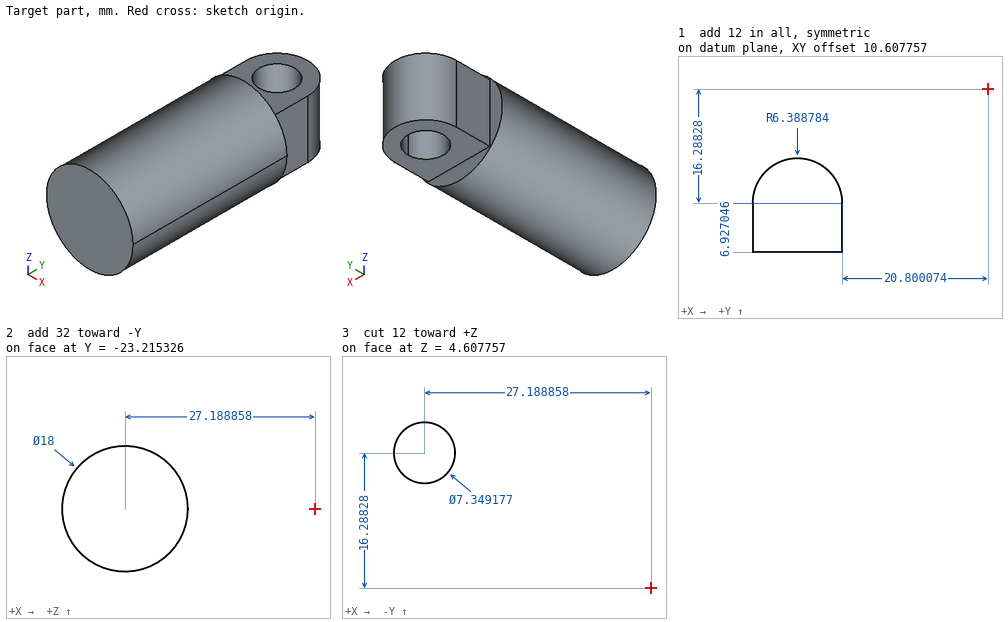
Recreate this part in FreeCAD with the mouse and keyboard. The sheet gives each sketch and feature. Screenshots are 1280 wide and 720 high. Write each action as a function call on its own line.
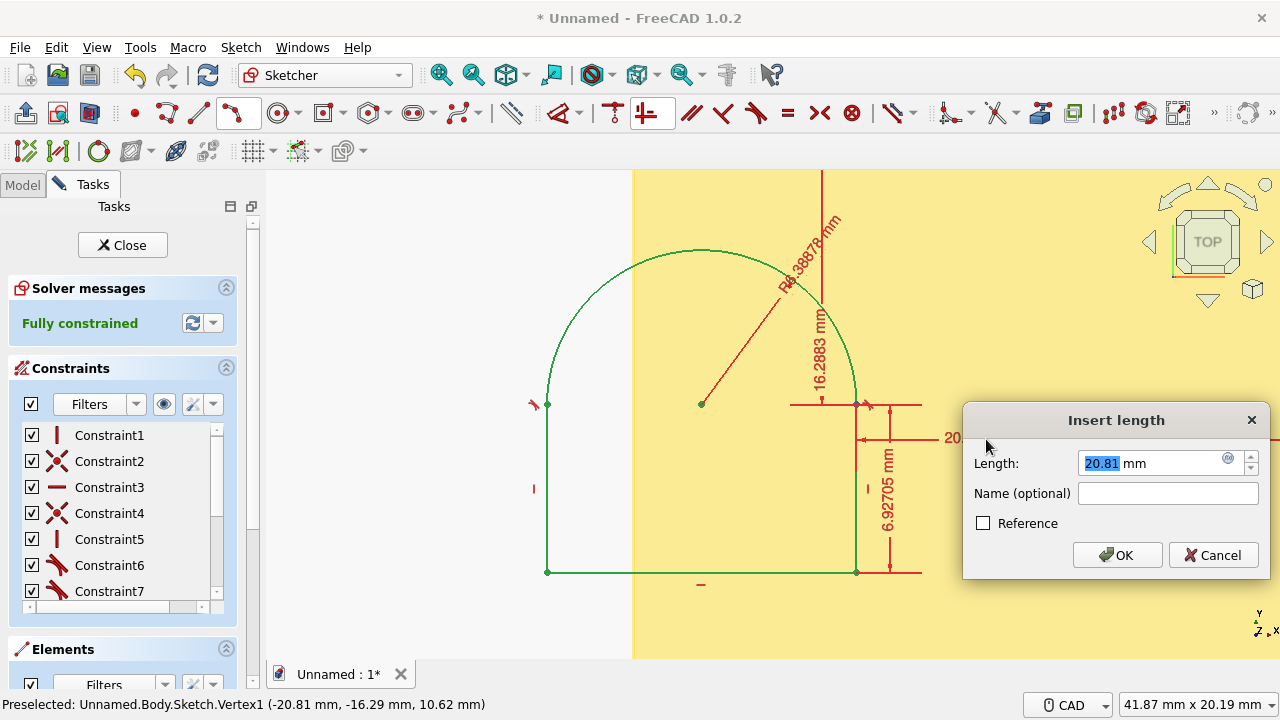
text(20.800074)
key(Return)
key(Escape)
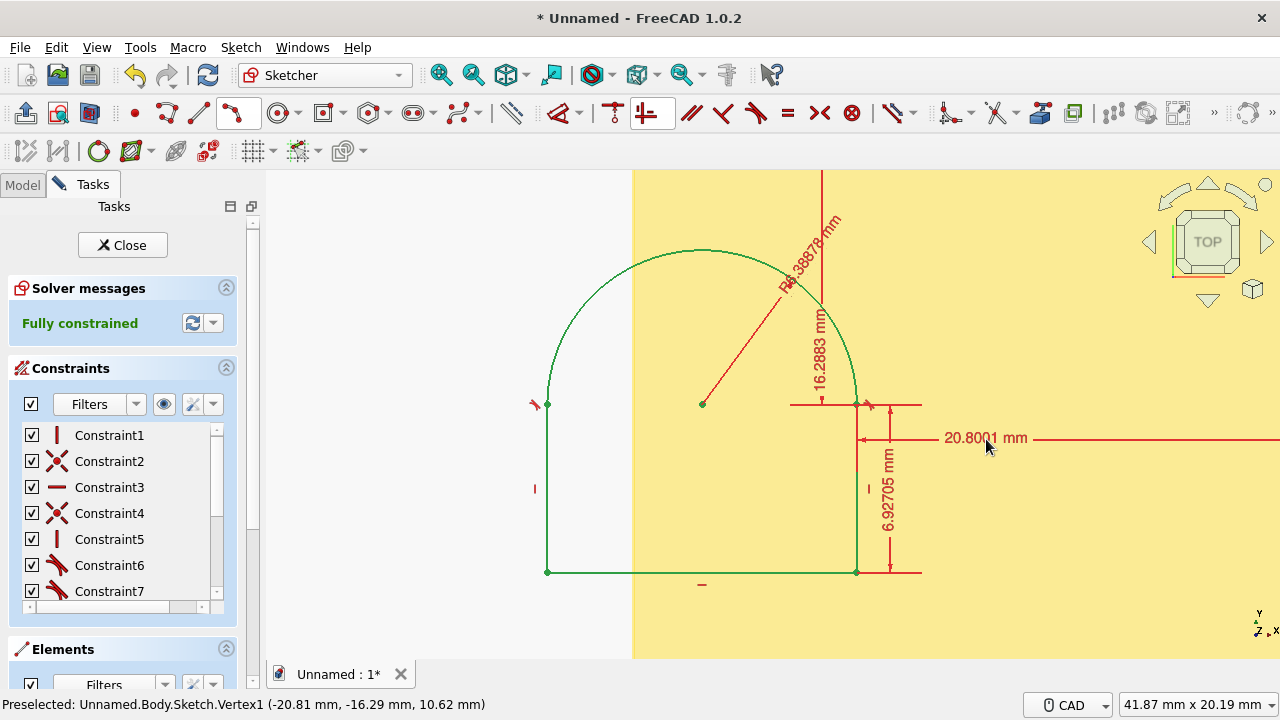
click(123, 245)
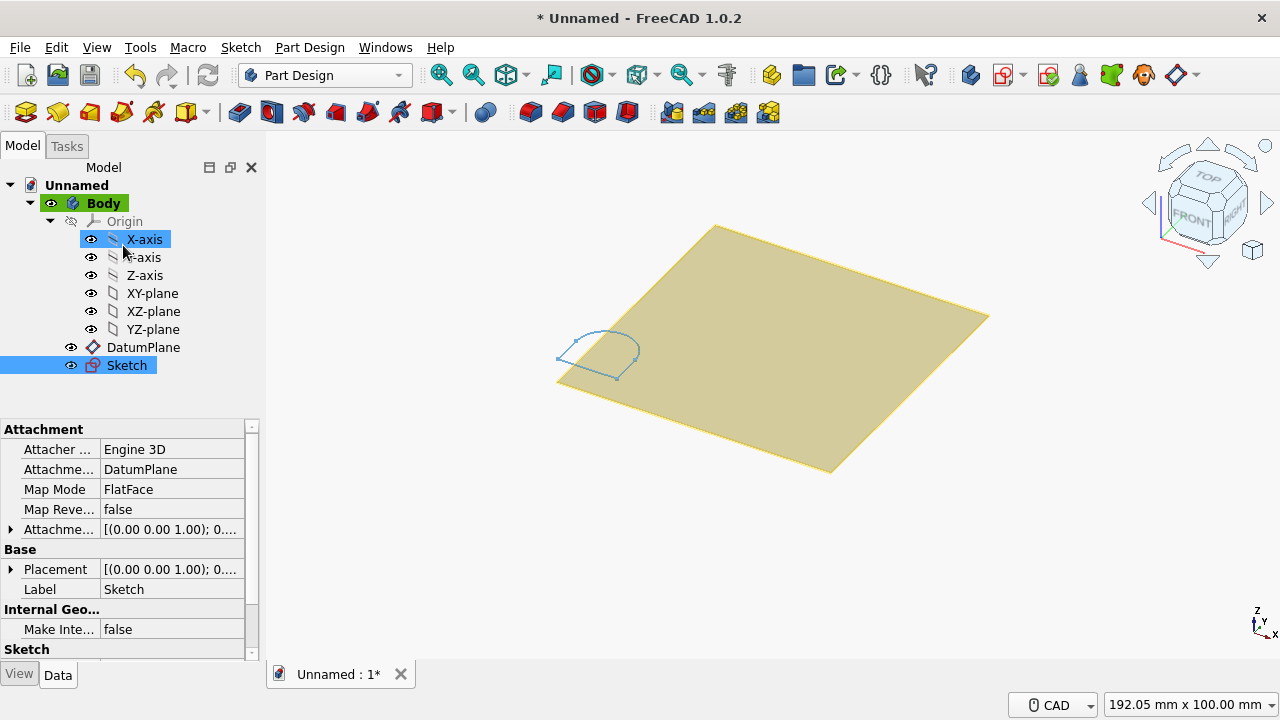
click(26, 112)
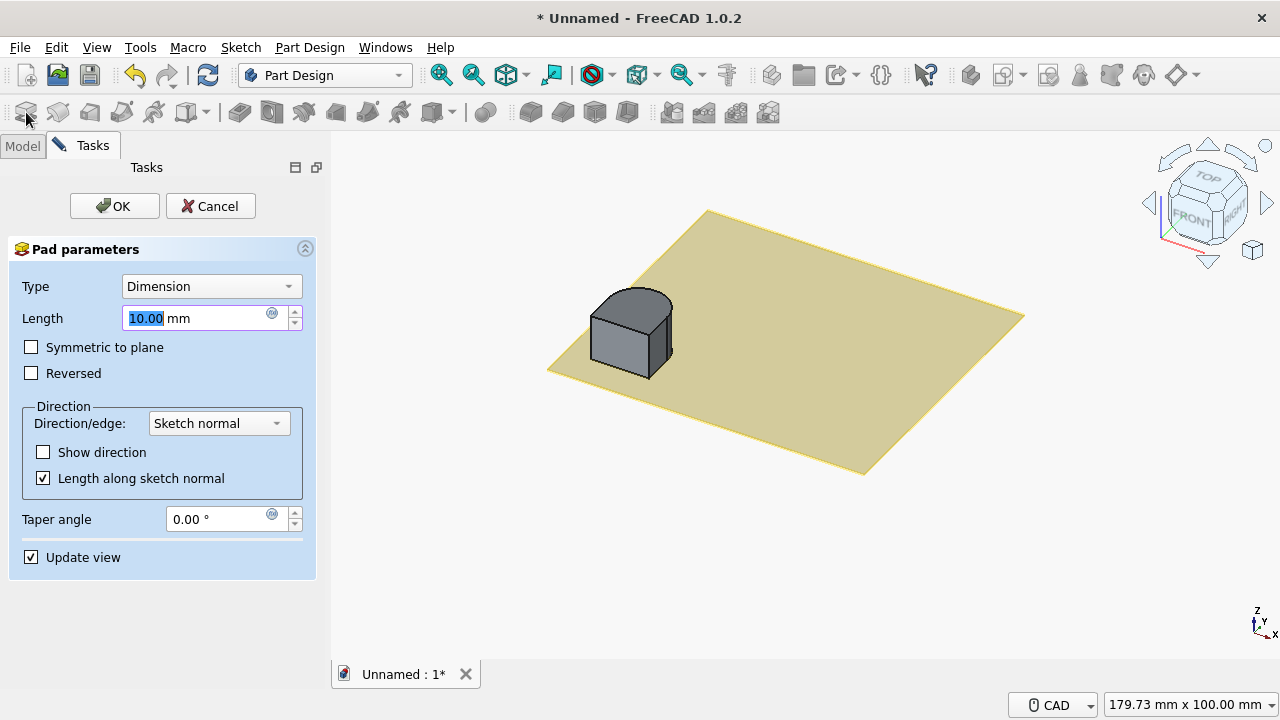
text(12)
key(Tab)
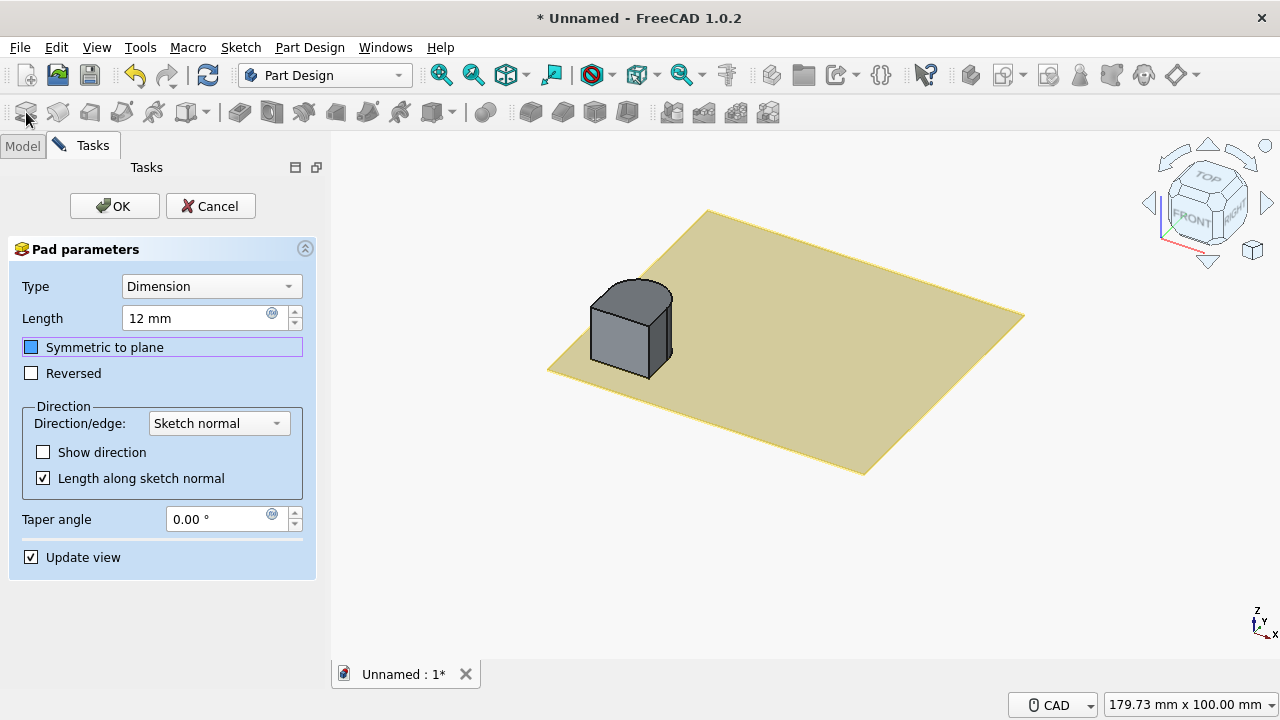
click(30, 347)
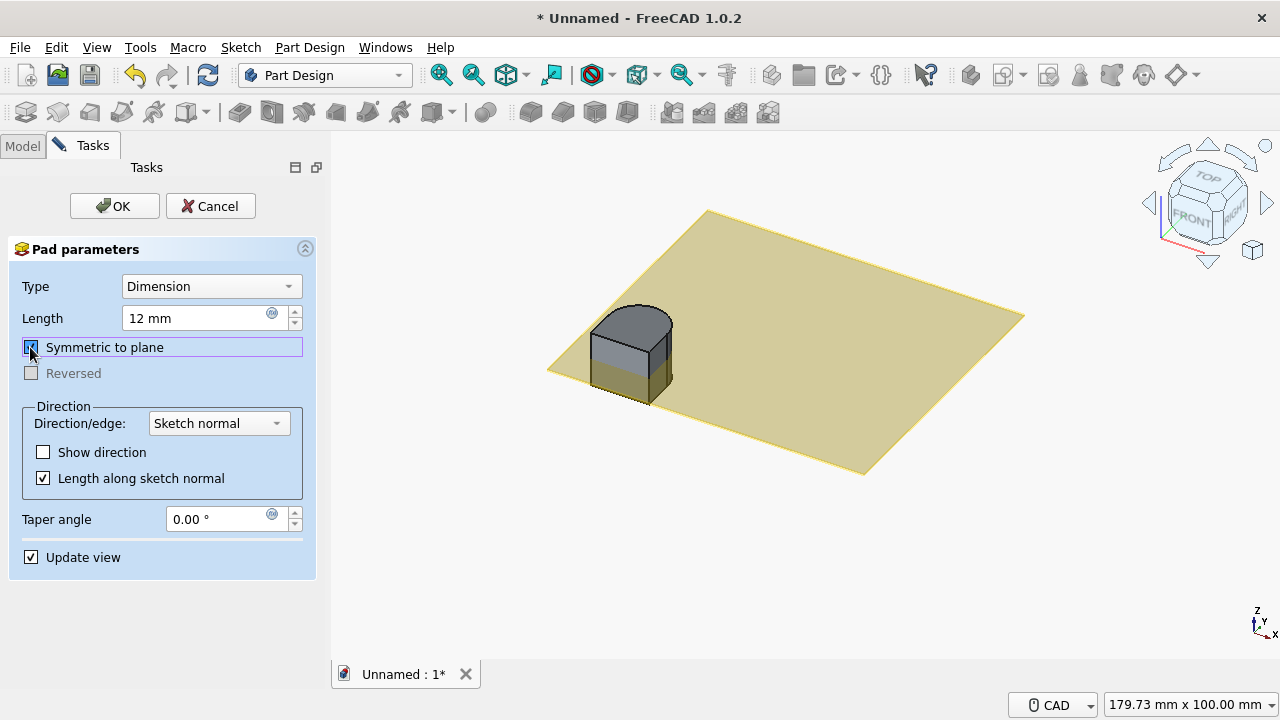
click(115, 206)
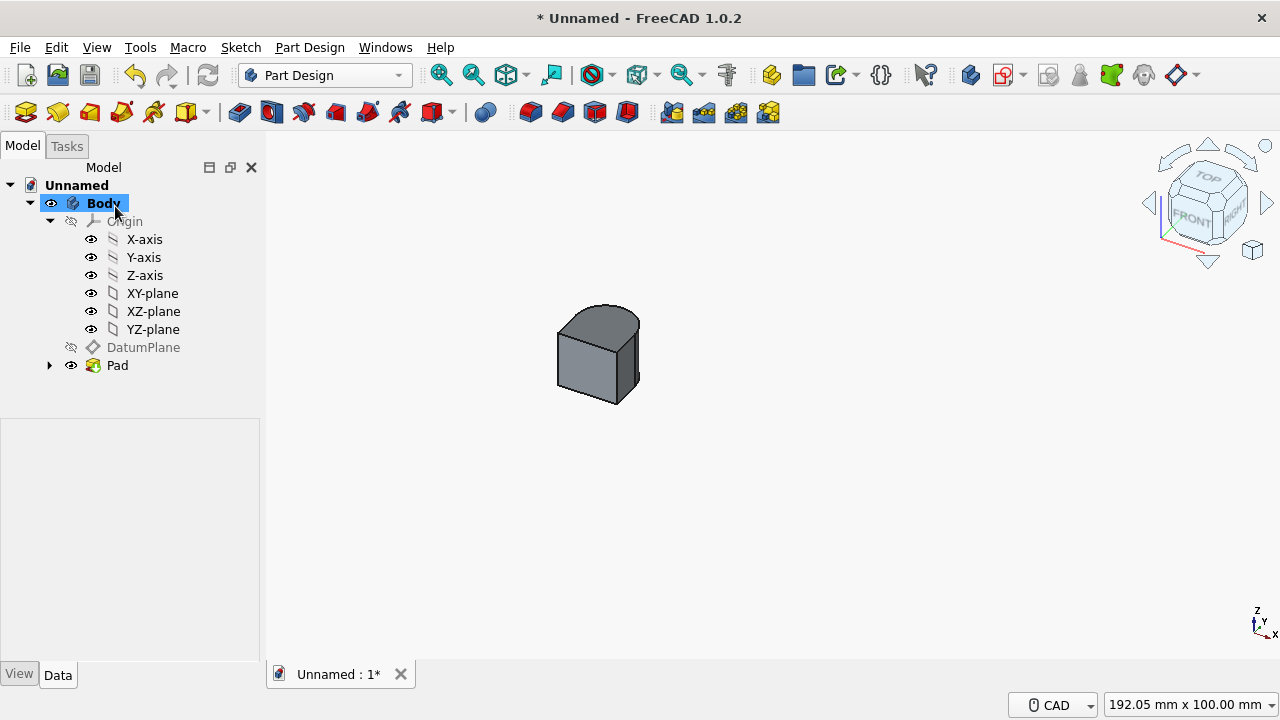
click(442, 76)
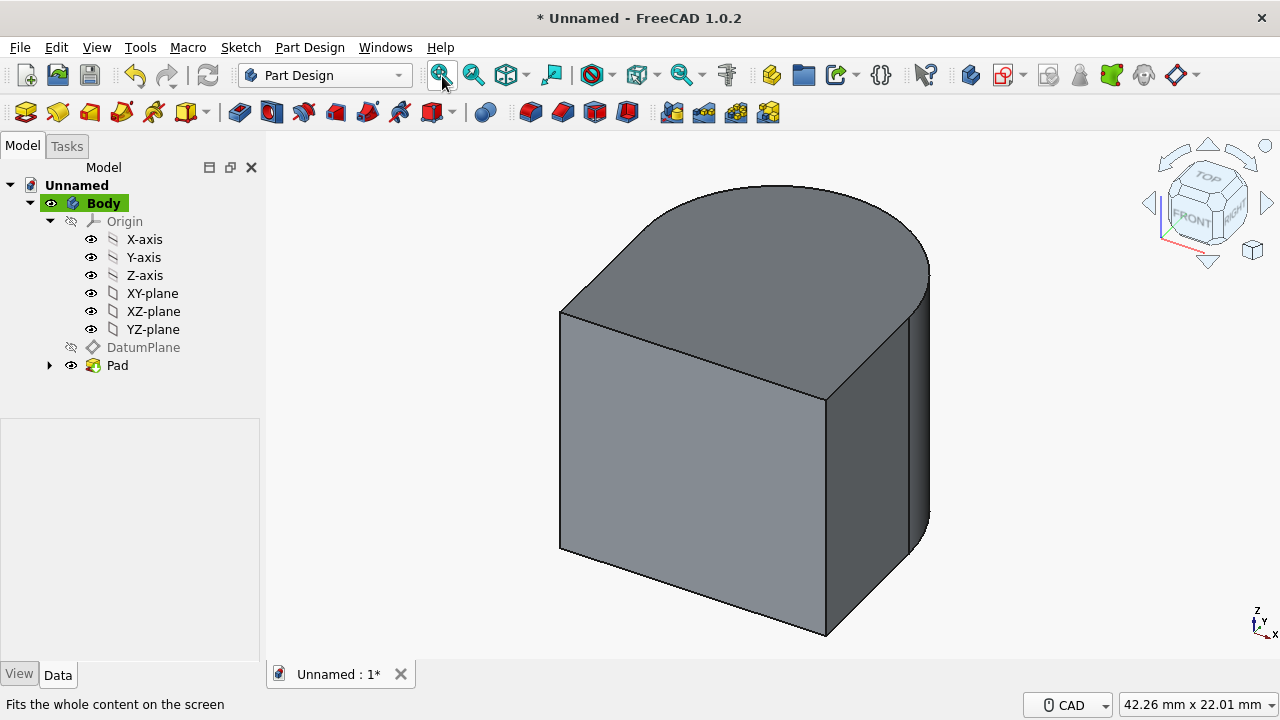
click(693, 473)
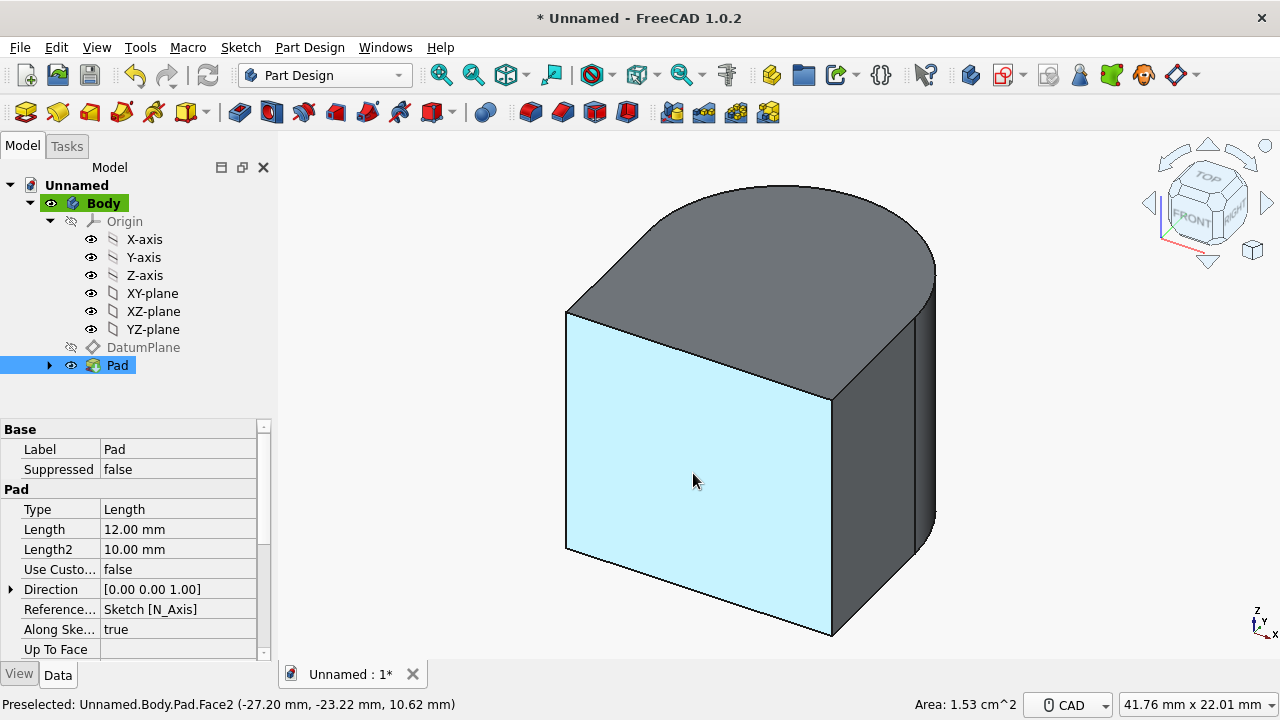
click(1004, 76)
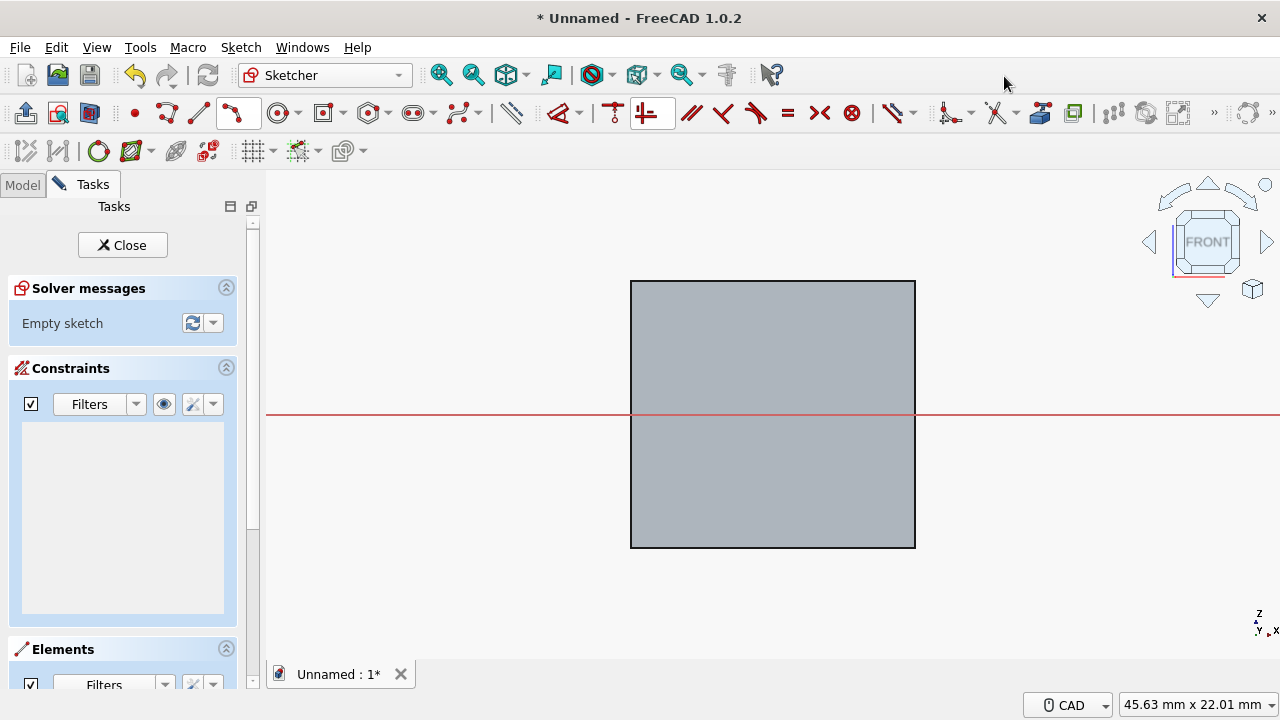
scroll(294, 414, down, 2)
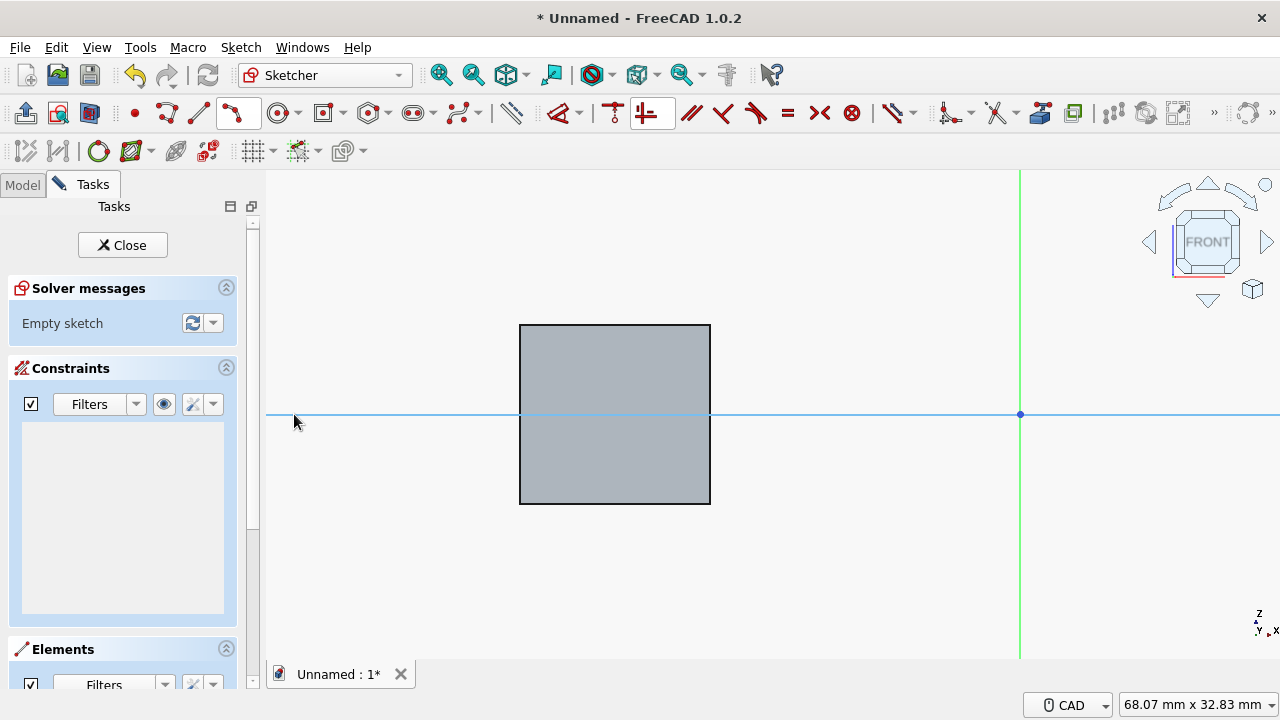
click(278, 114)